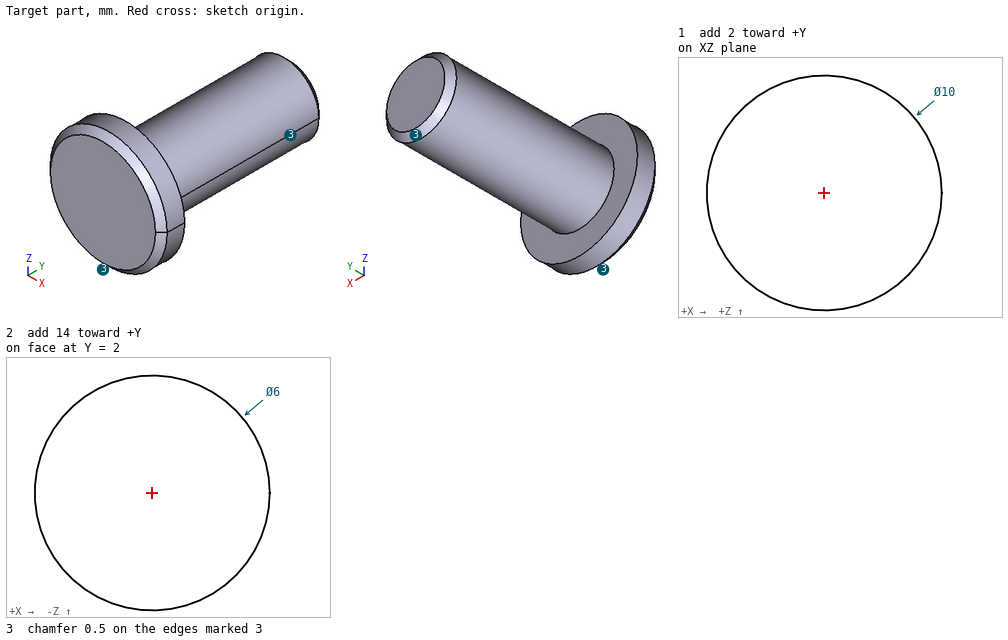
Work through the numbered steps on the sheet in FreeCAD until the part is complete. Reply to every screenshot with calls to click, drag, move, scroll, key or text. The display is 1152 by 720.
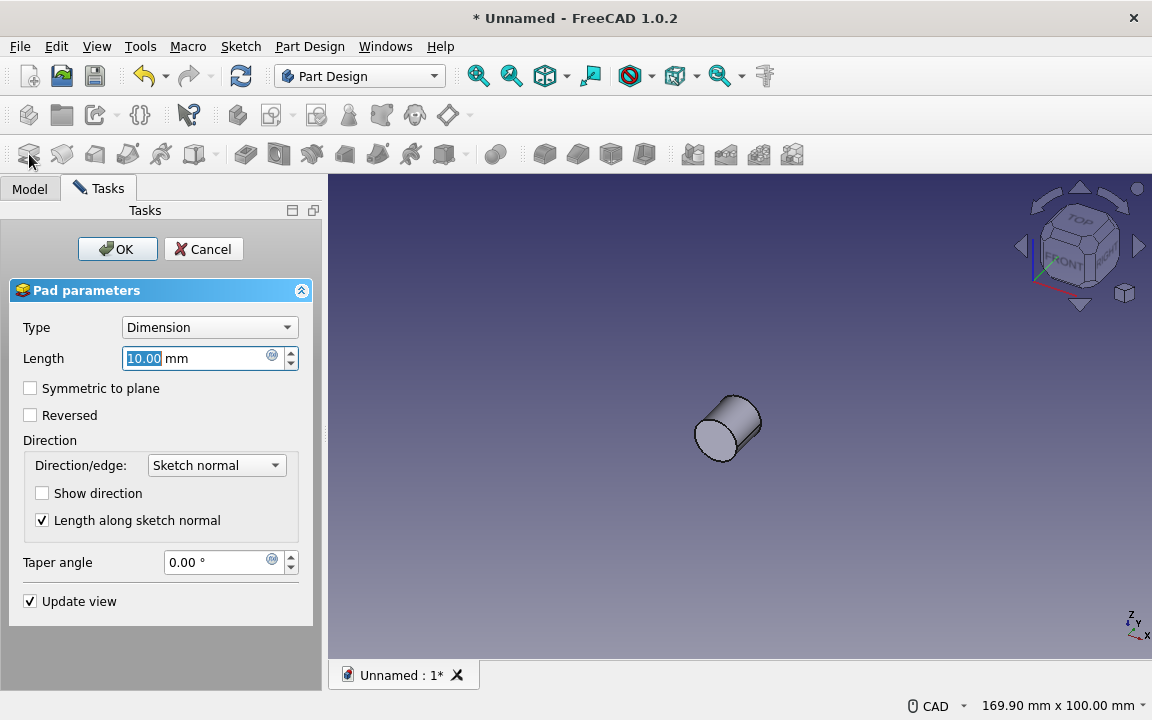
text(2)
key(Tab)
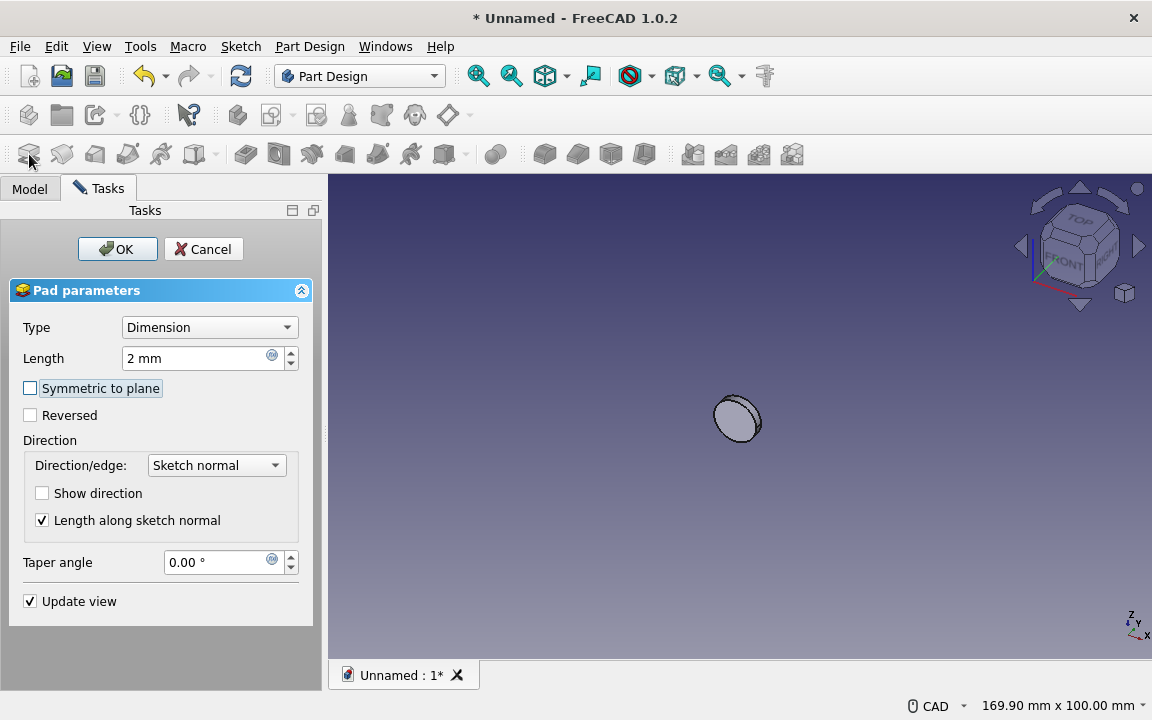
click(31, 415)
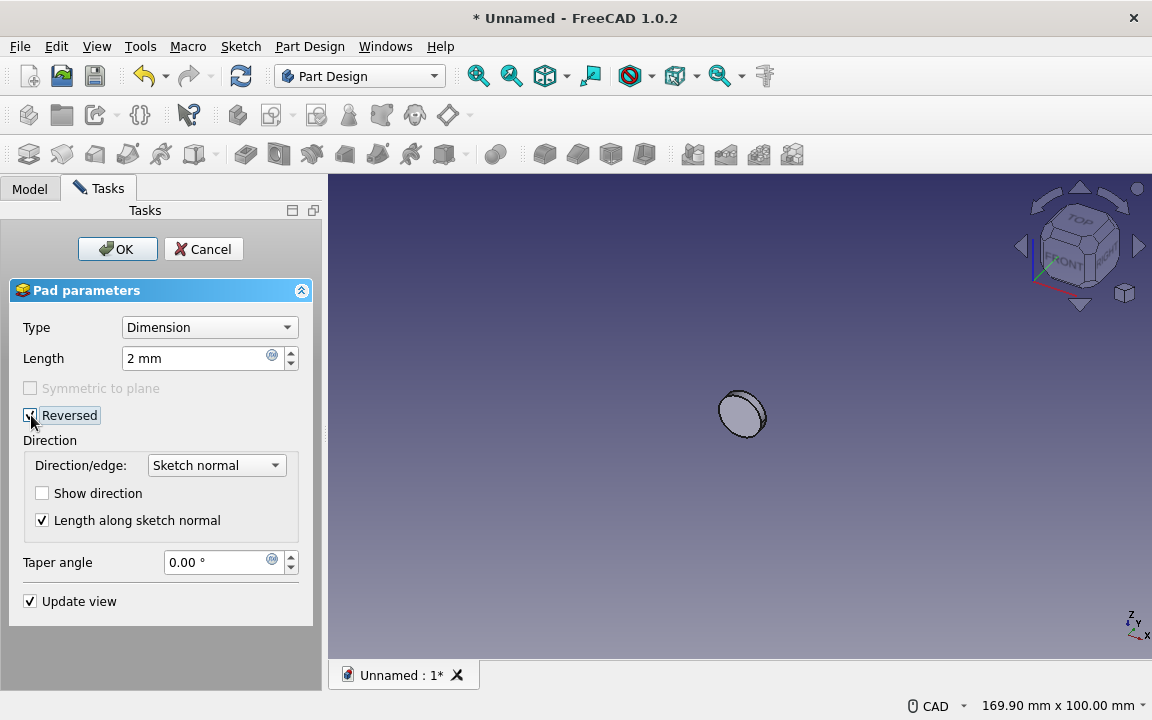
click(118, 249)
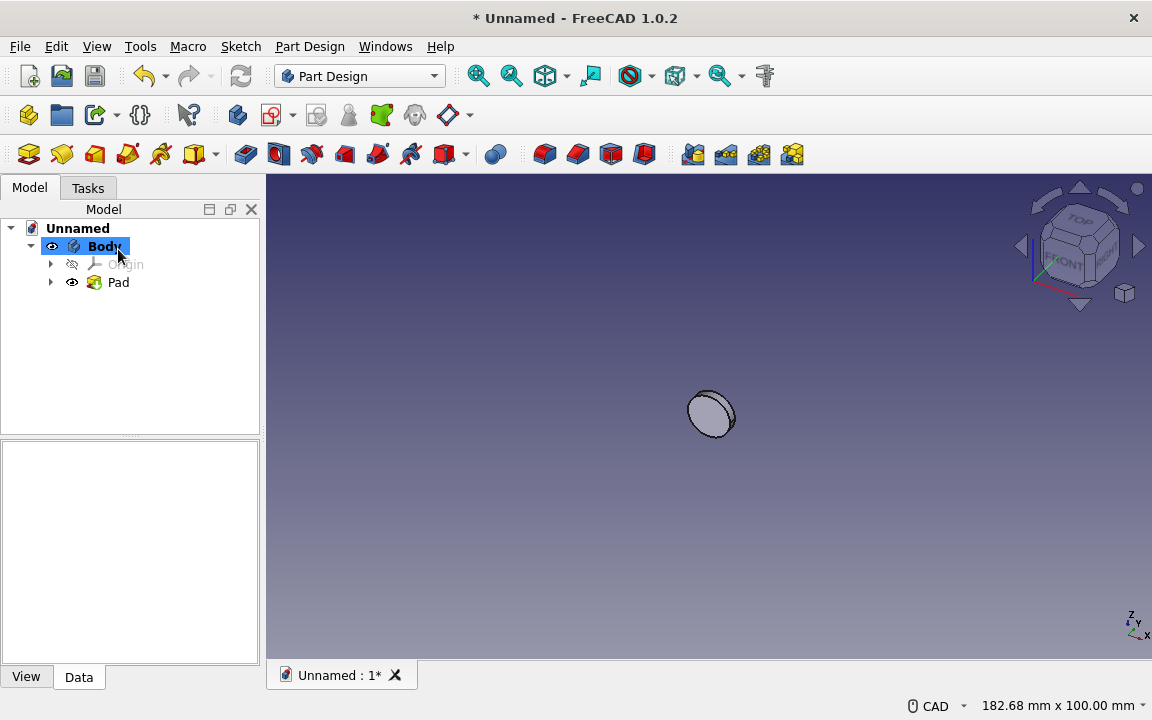
key(v)
key(f)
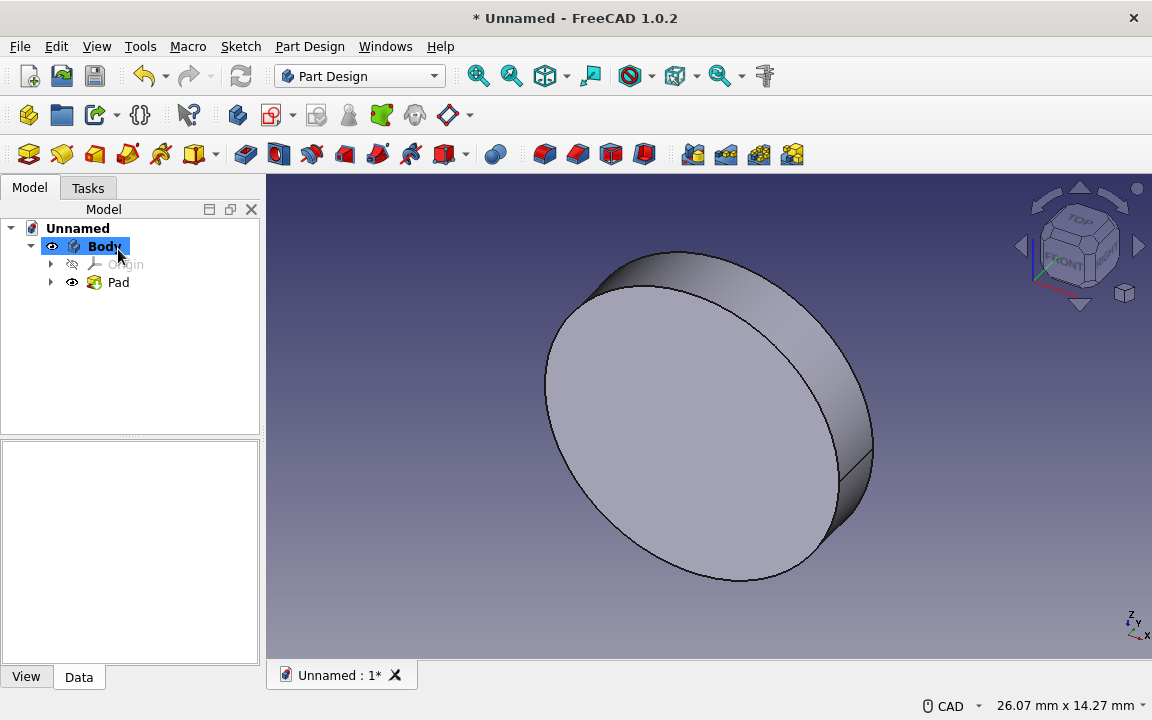
key(4)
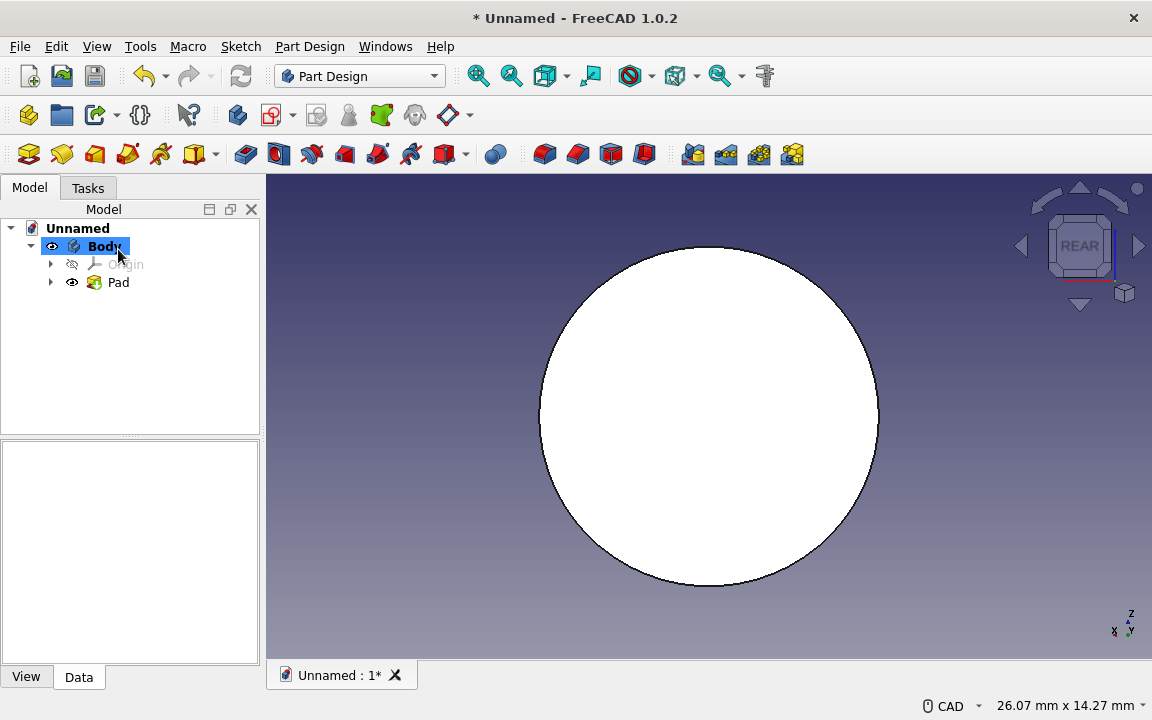
click(709, 416)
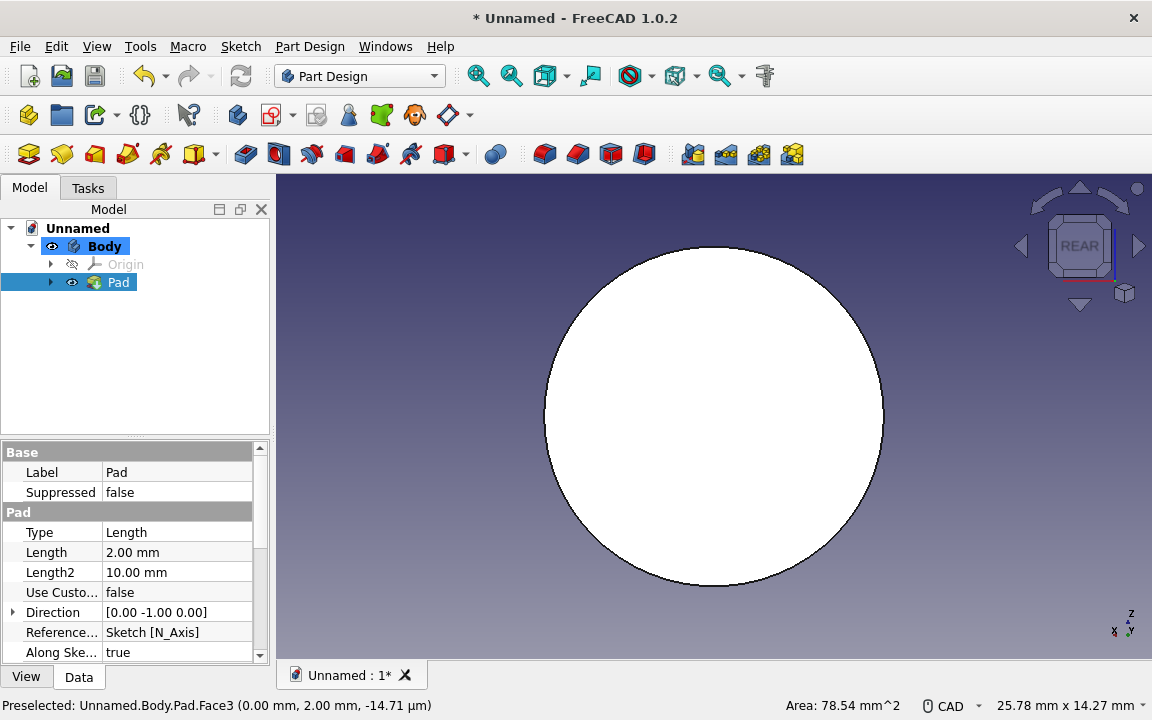
click(270, 116)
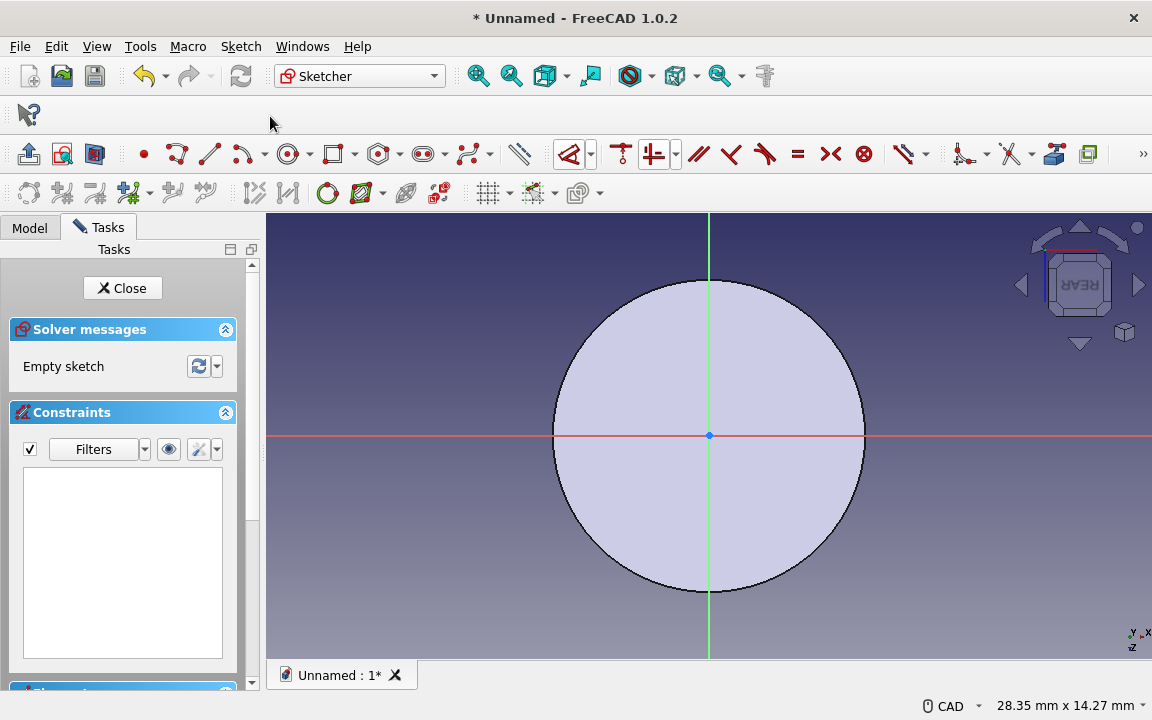
scroll(848, 436, up, 2)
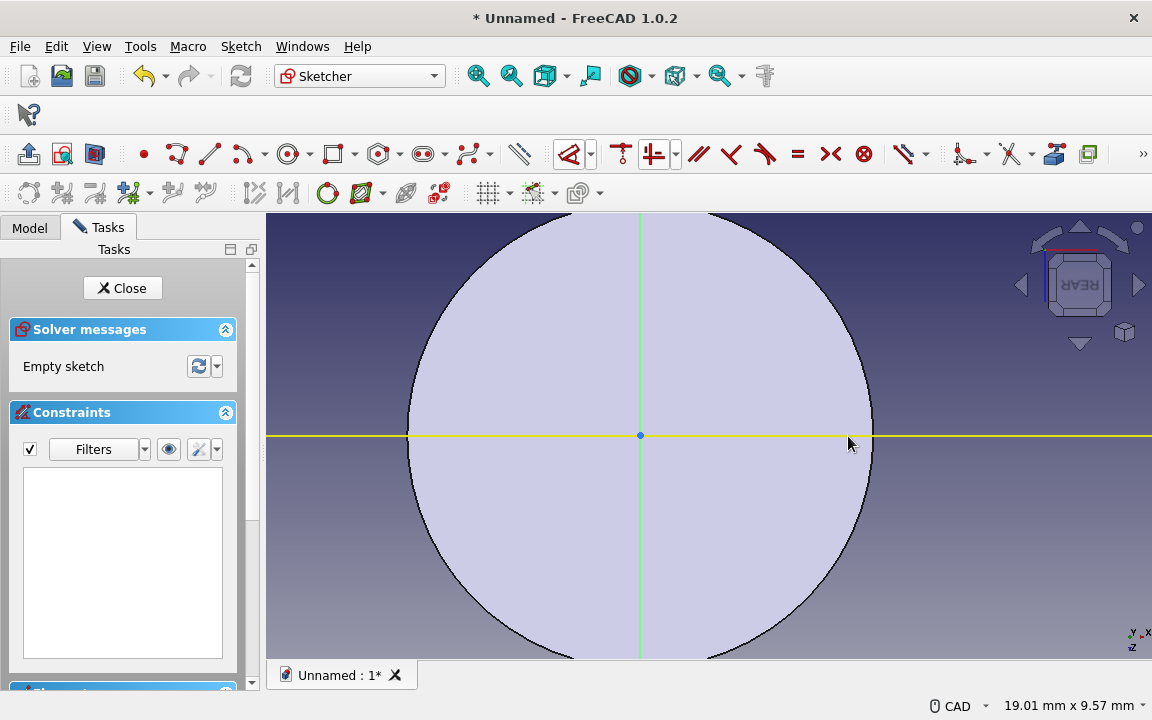
key(g)
key(c)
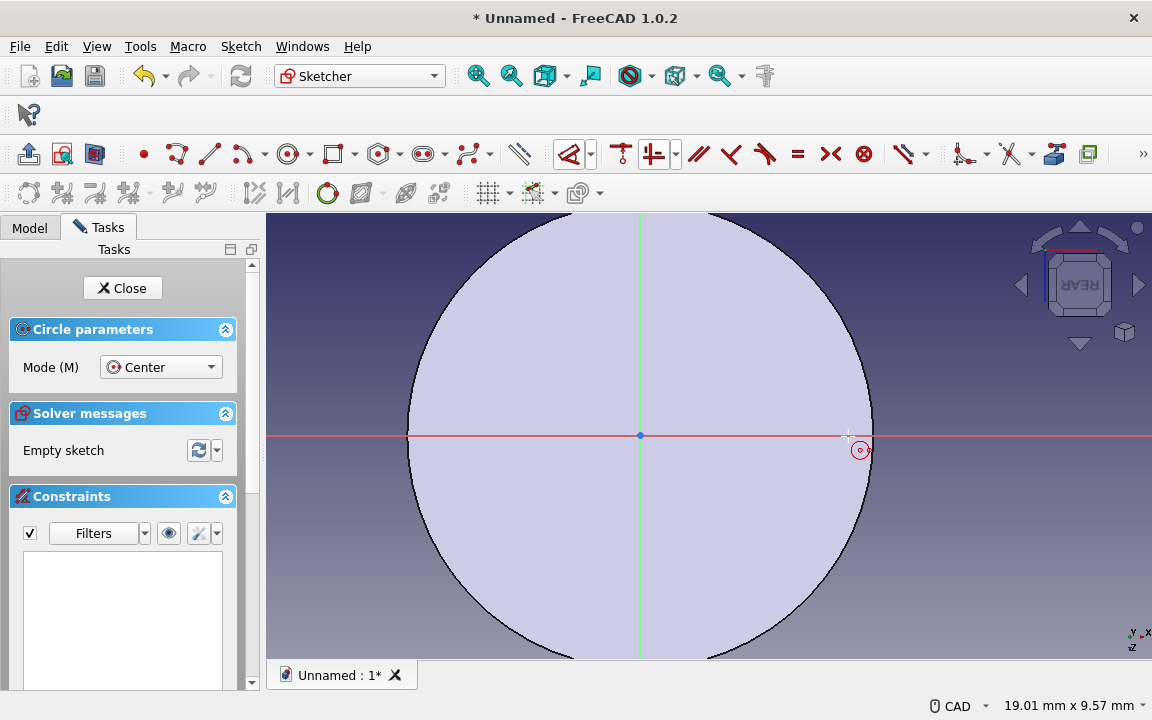
click(640, 436)
click(739, 337)
key(Escape)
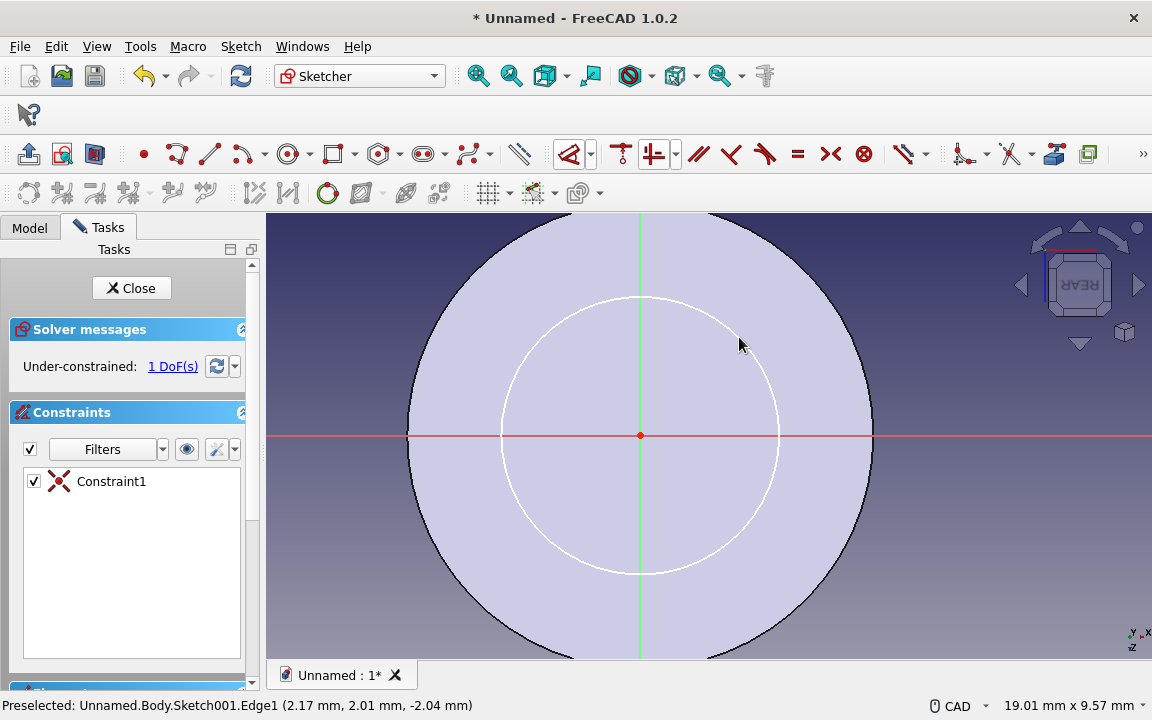
key(d)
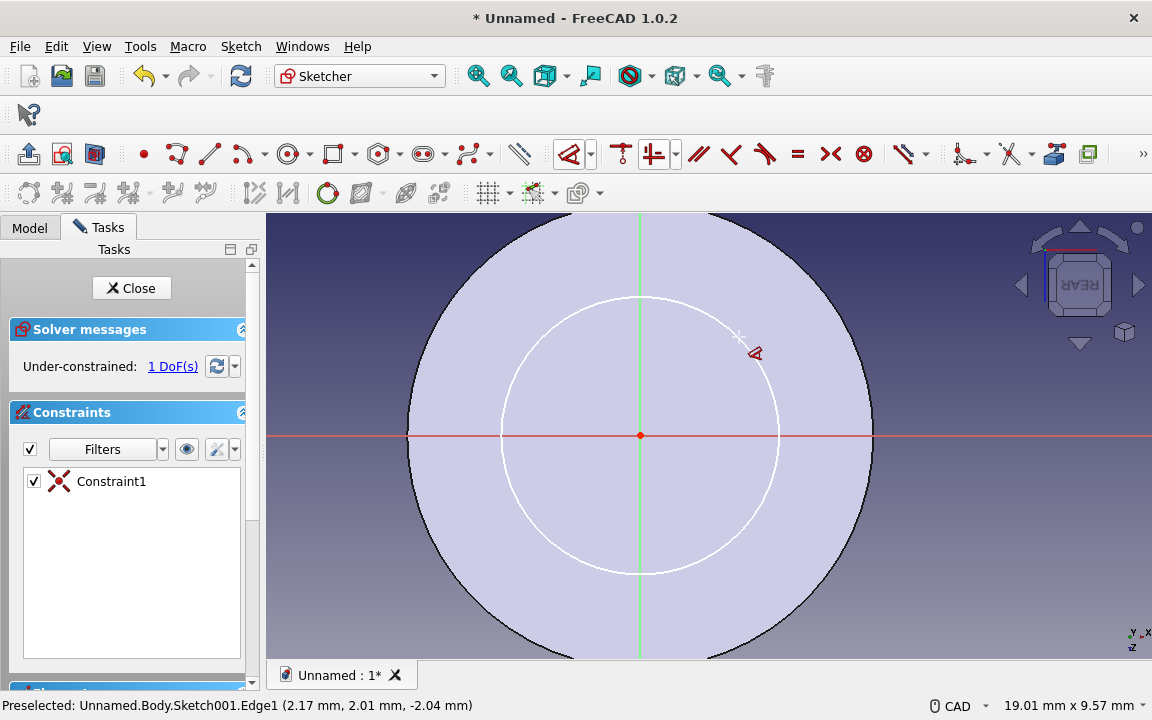
click(738, 337)
click(761, 314)